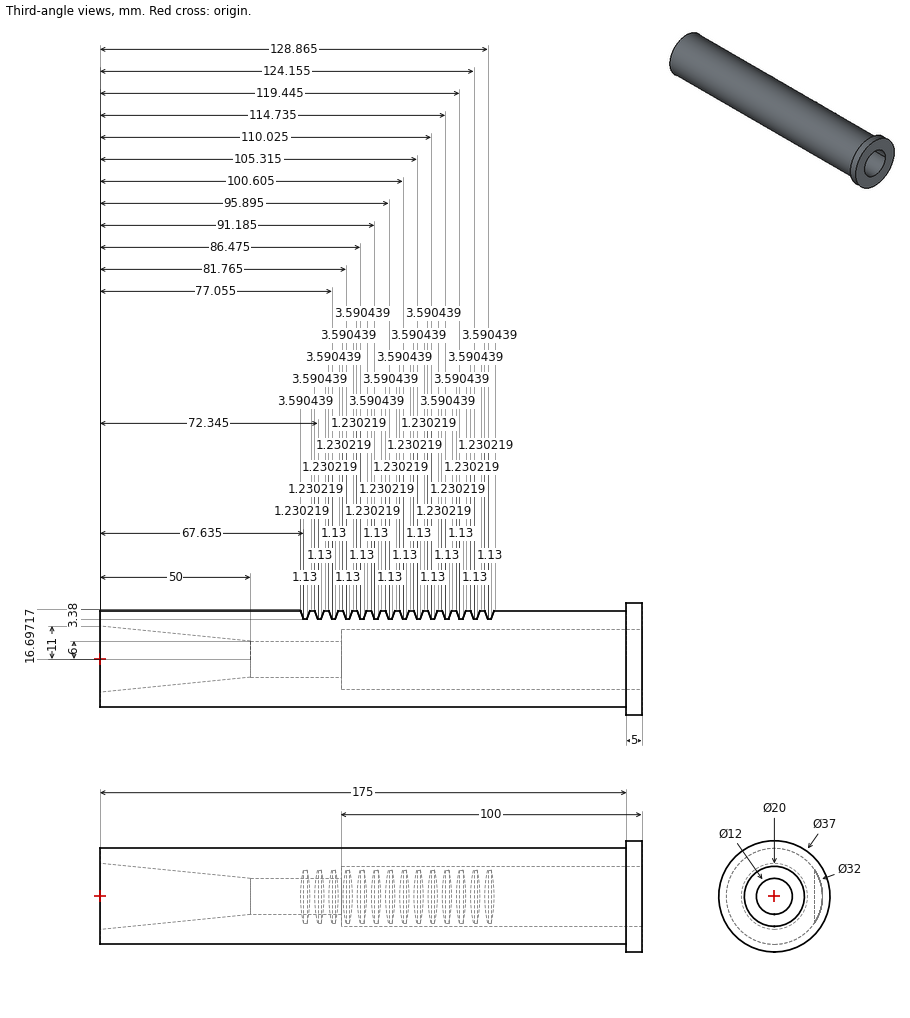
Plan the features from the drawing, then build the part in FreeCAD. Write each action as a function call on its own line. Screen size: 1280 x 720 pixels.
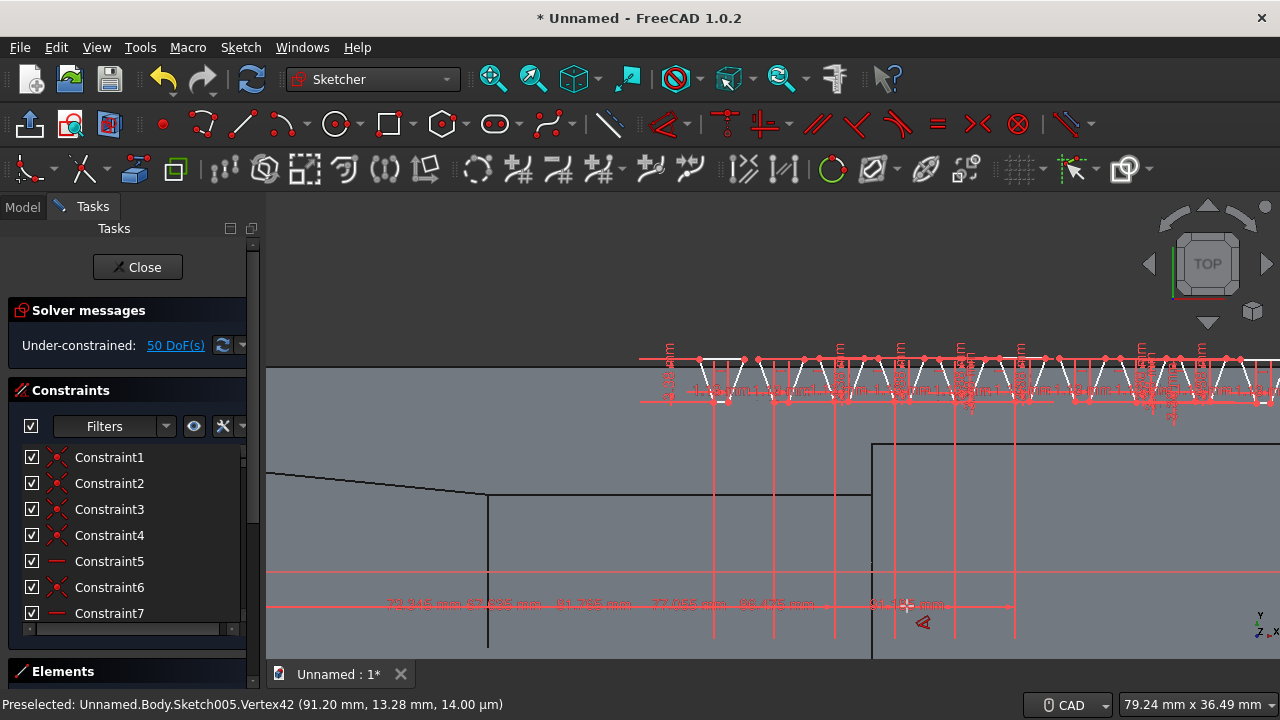
click(1075, 402)
click(505, 368)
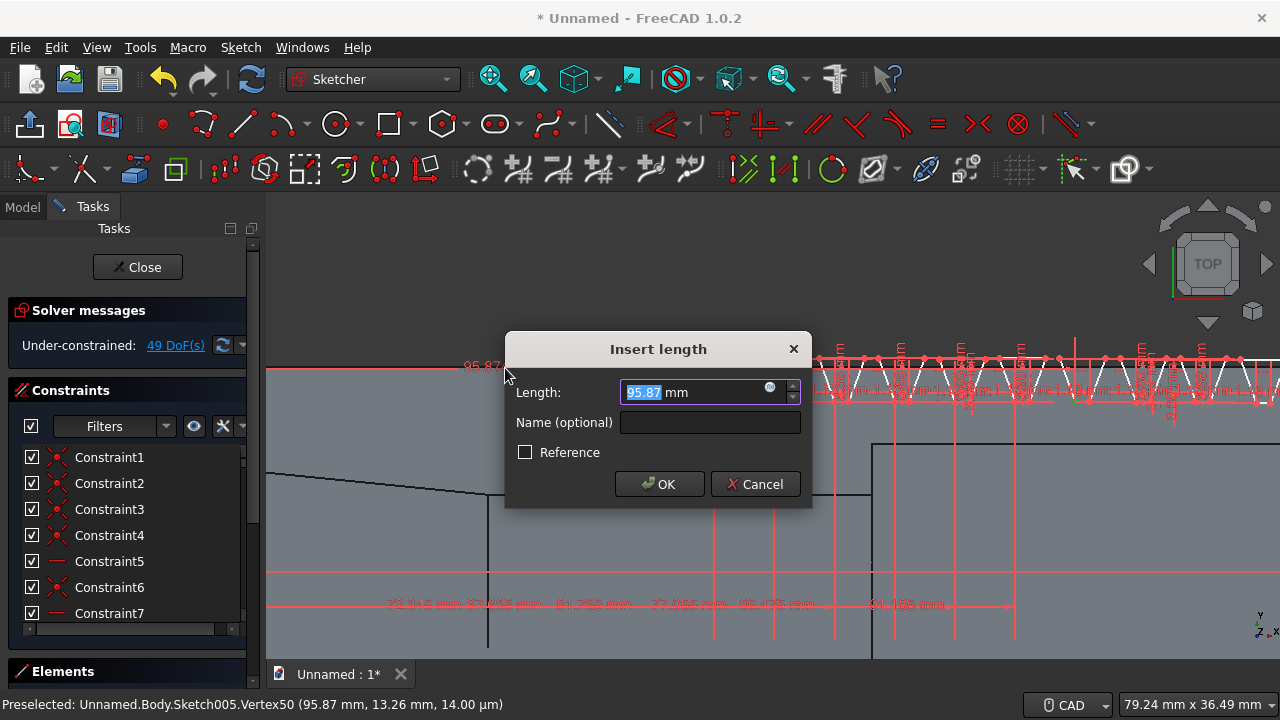
text(95.895)
key(Return)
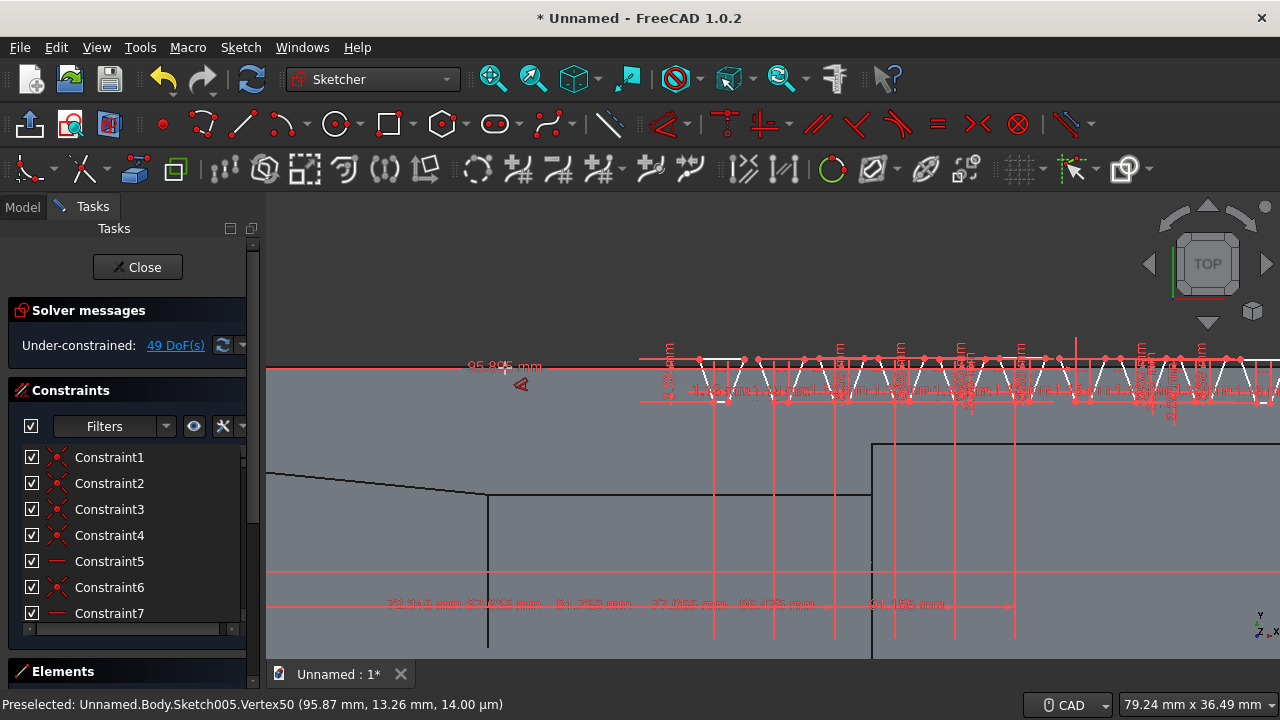
click(731, 359)
click(722, 325)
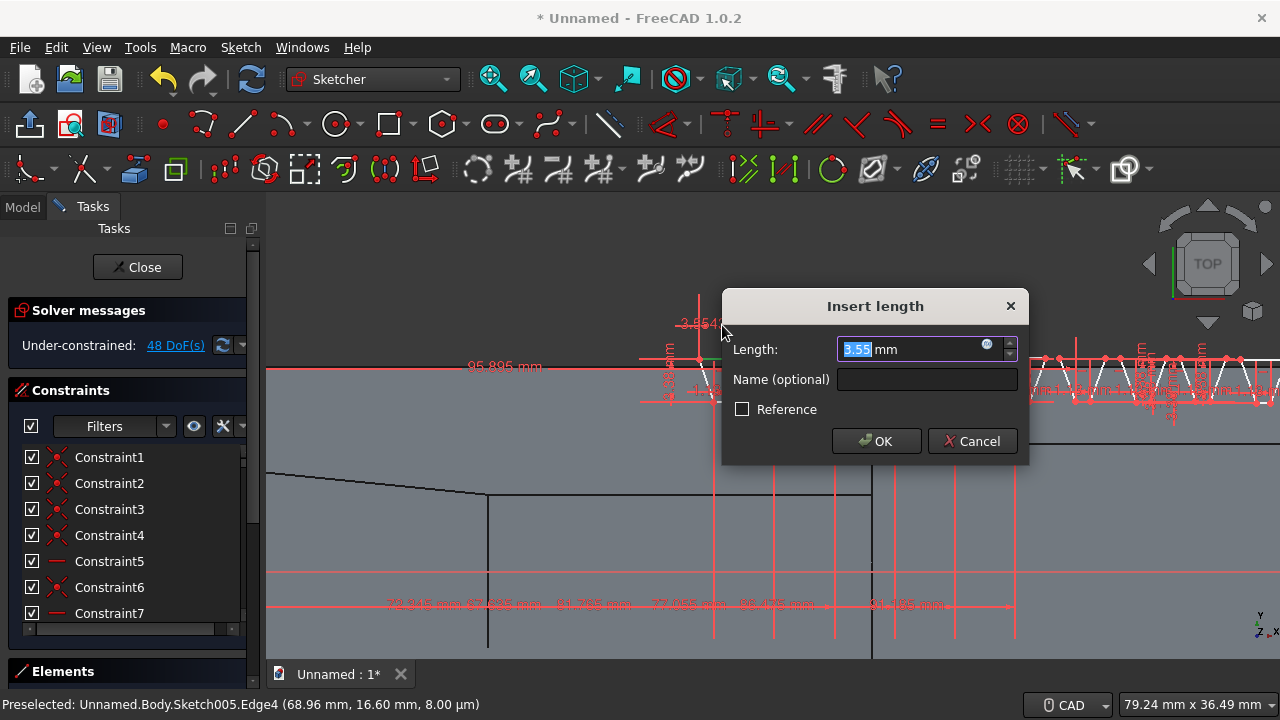
text(3.590439)
key(Return)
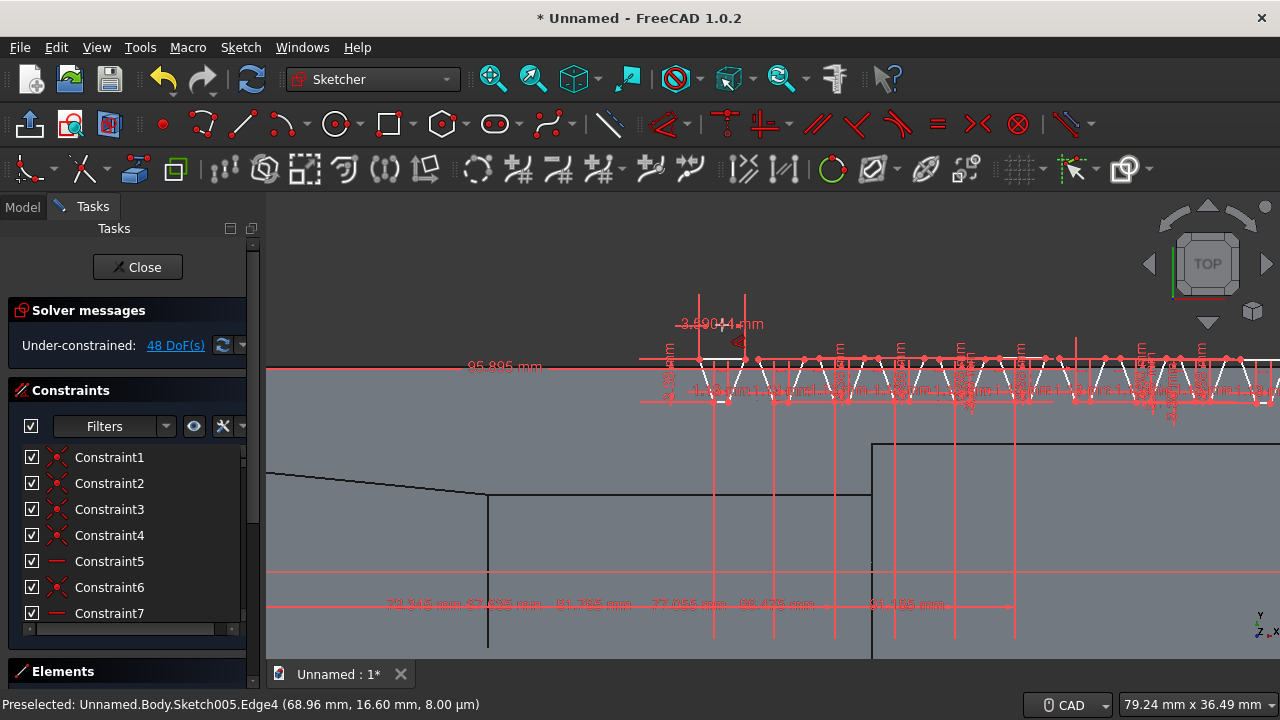
click(791, 359)
click(792, 325)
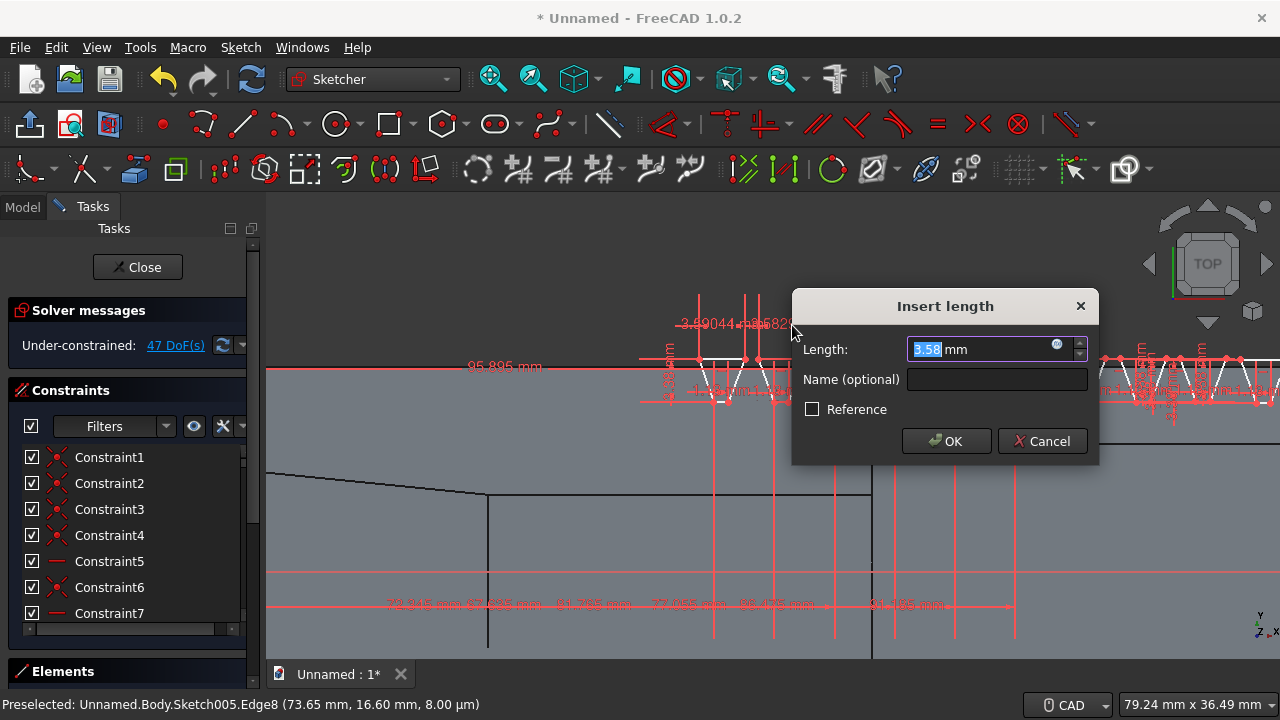
text(3.590439)
key(Return)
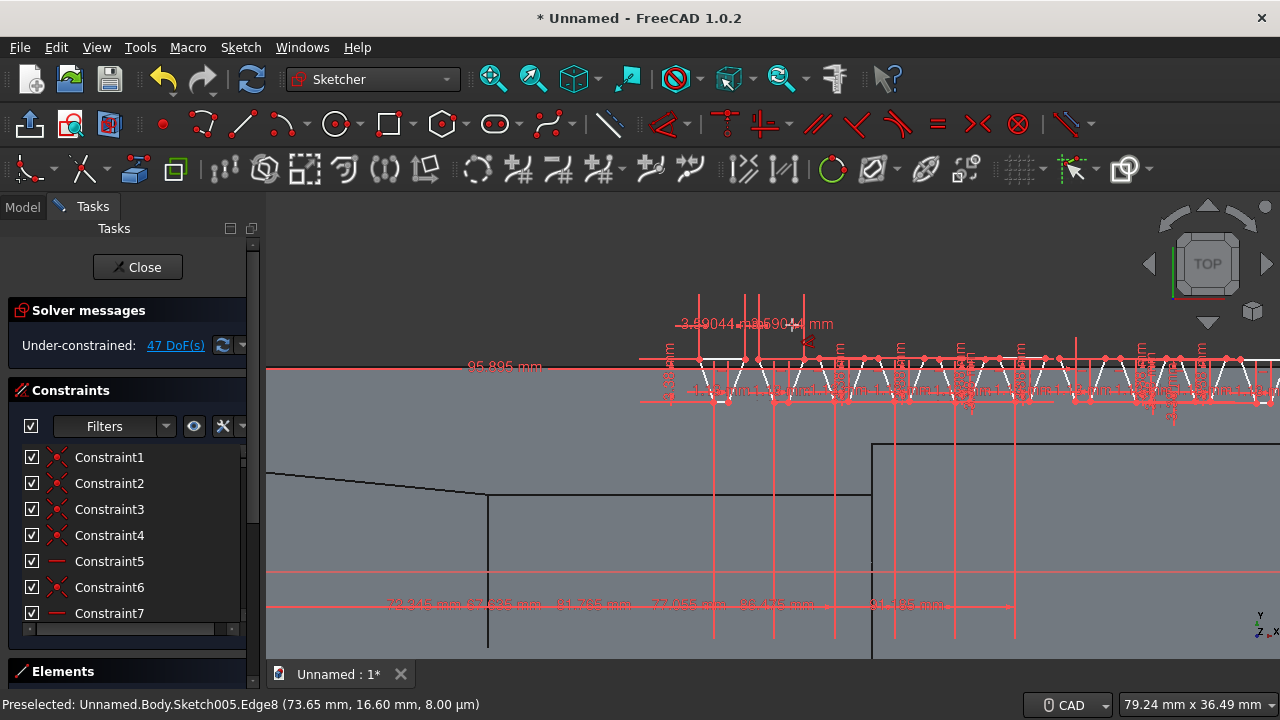
click(851, 358)
click(842, 300)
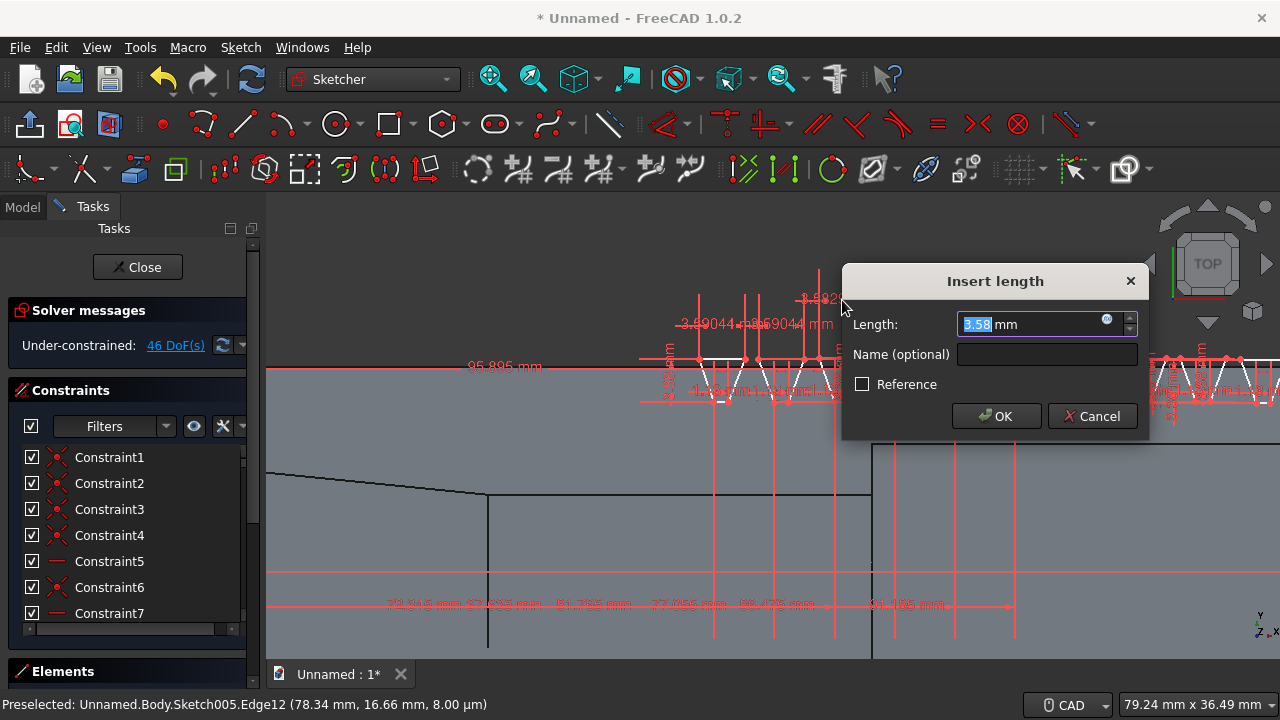
text(3.590439)
key(Return)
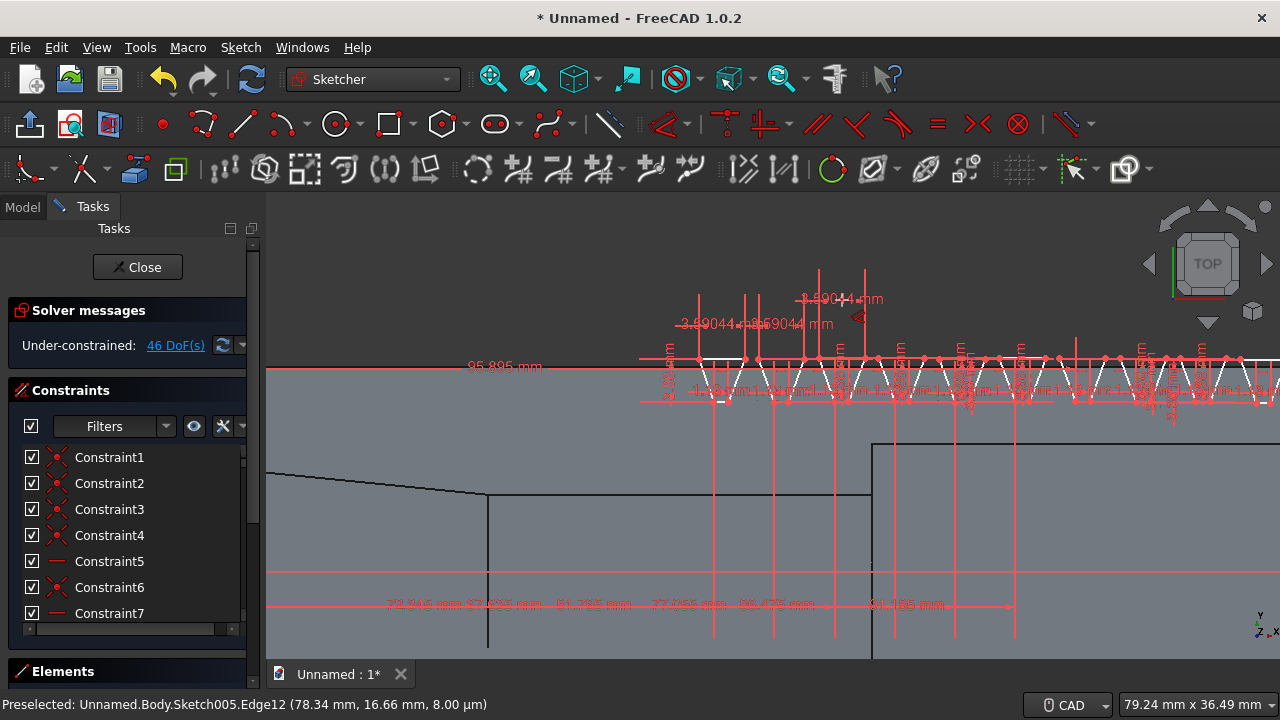
click(911, 358)
click(902, 324)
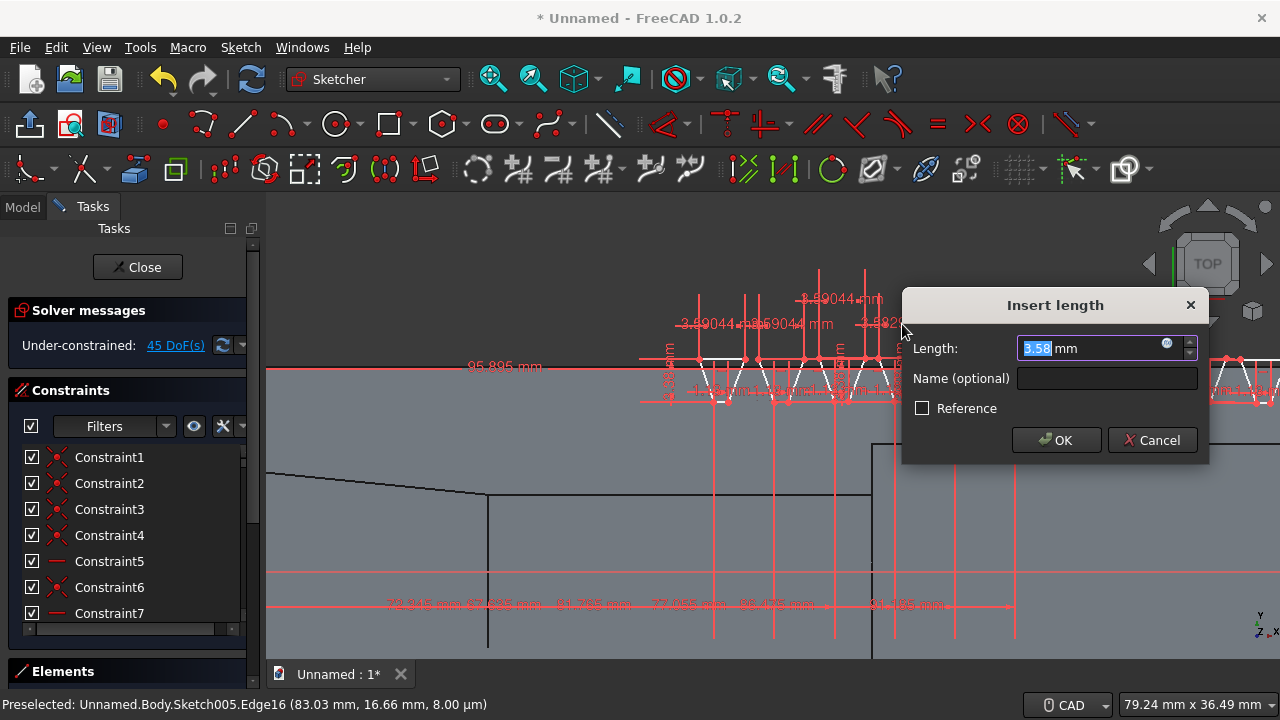
text(3.590439)
key(Return)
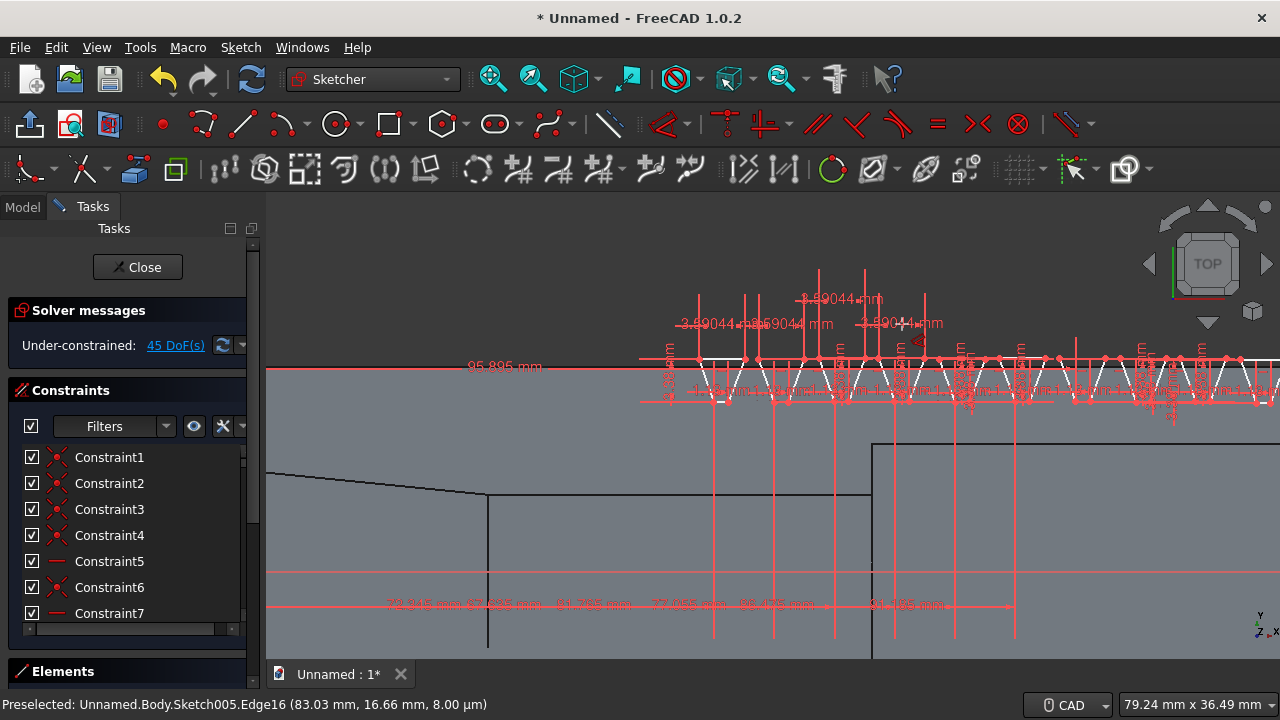
click(972, 359)
click(973, 325)